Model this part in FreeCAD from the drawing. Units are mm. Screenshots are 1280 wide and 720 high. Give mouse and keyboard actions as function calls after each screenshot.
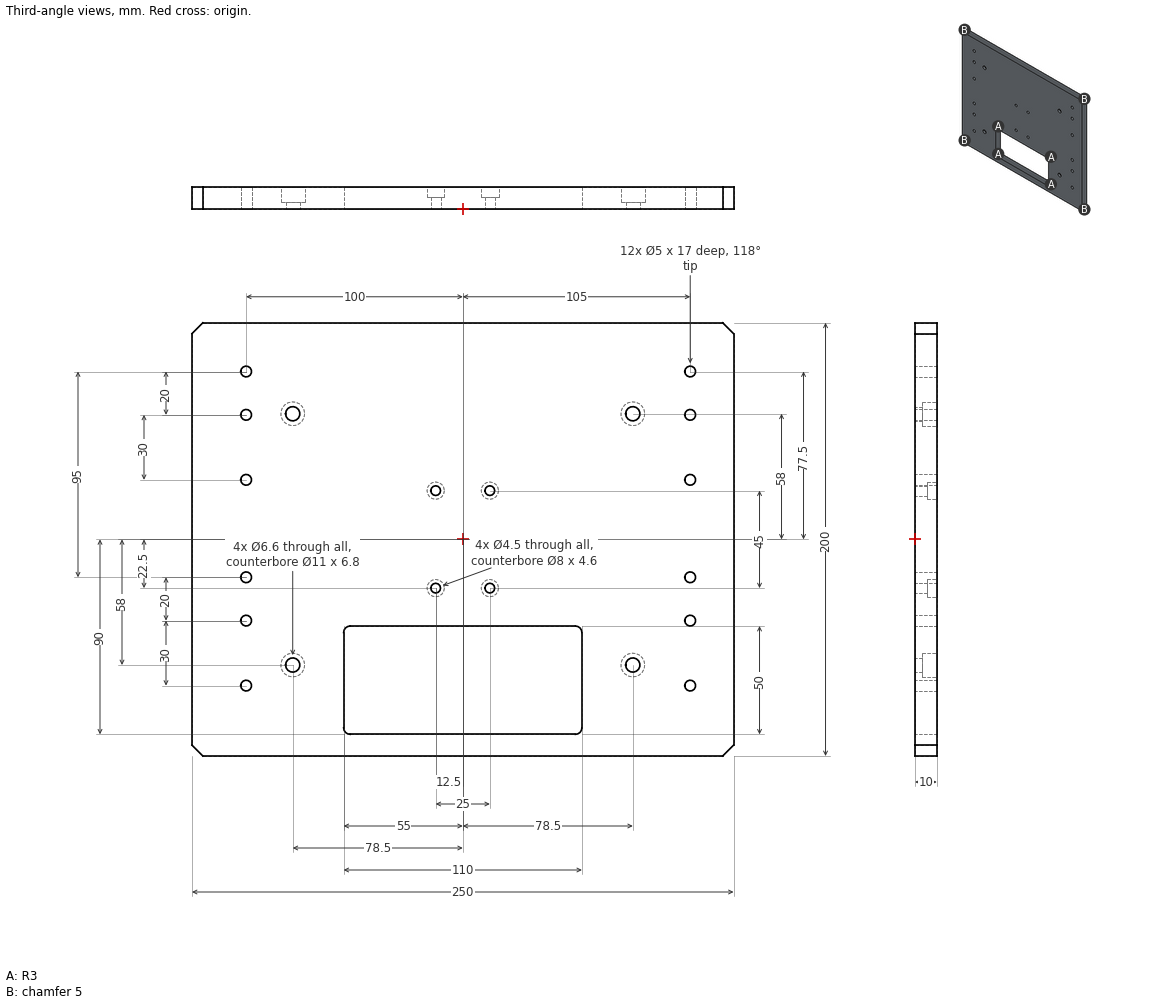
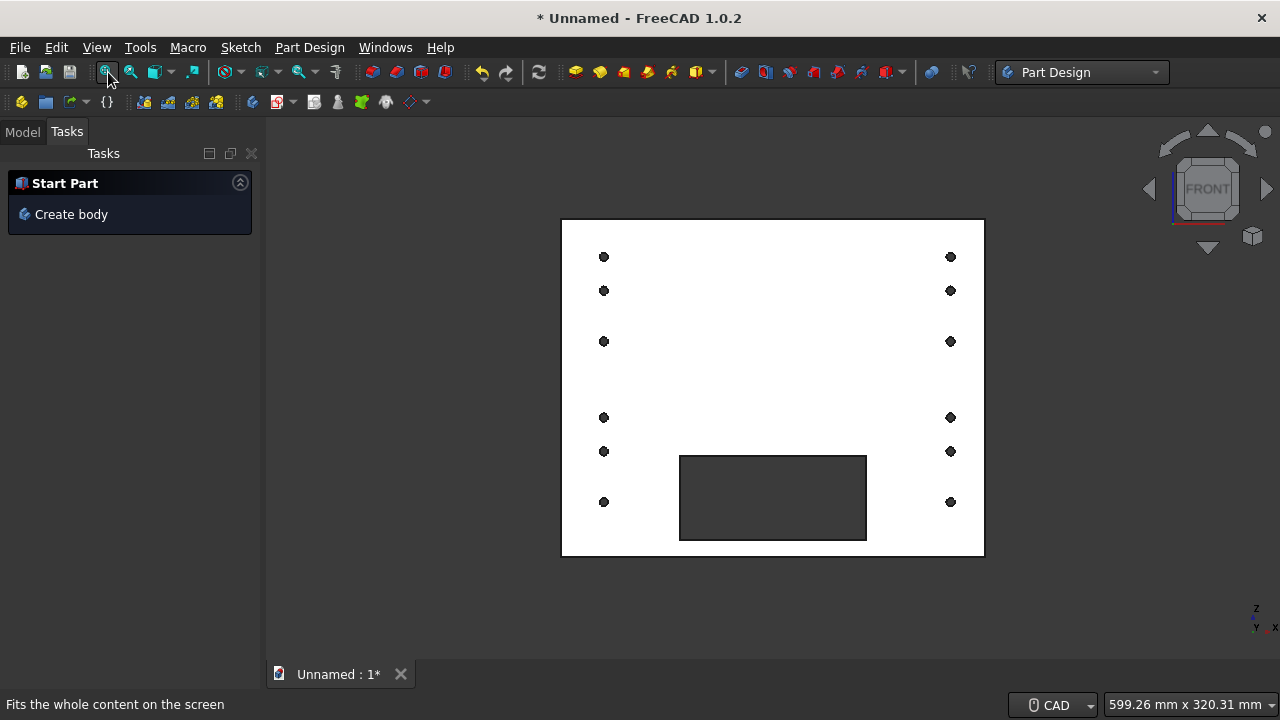
key(3)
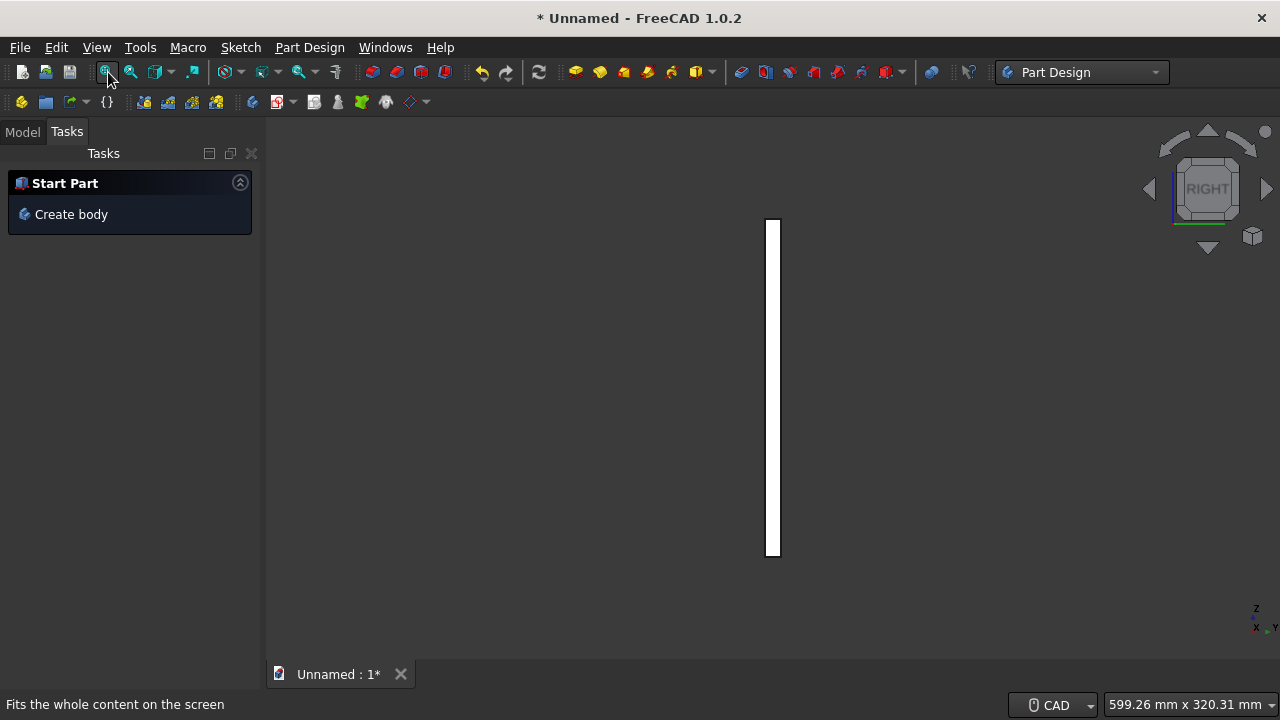
scroll(773, 455, up, 5)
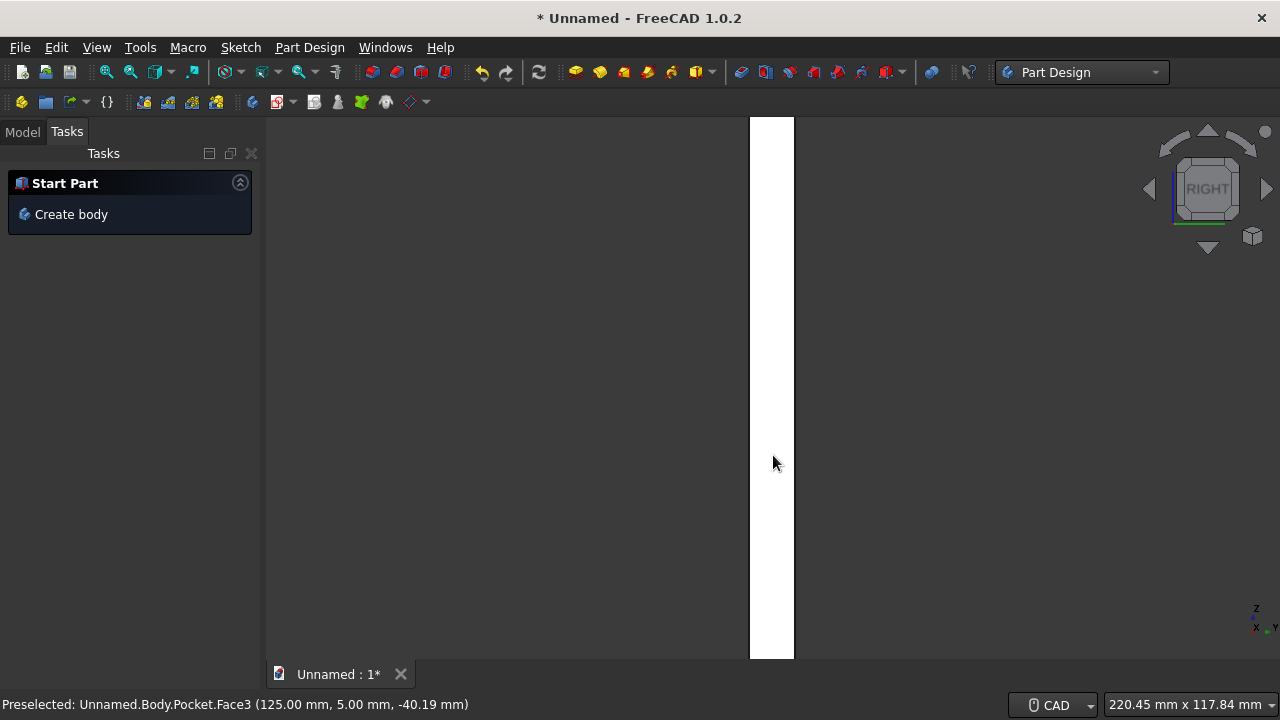
click(108, 72)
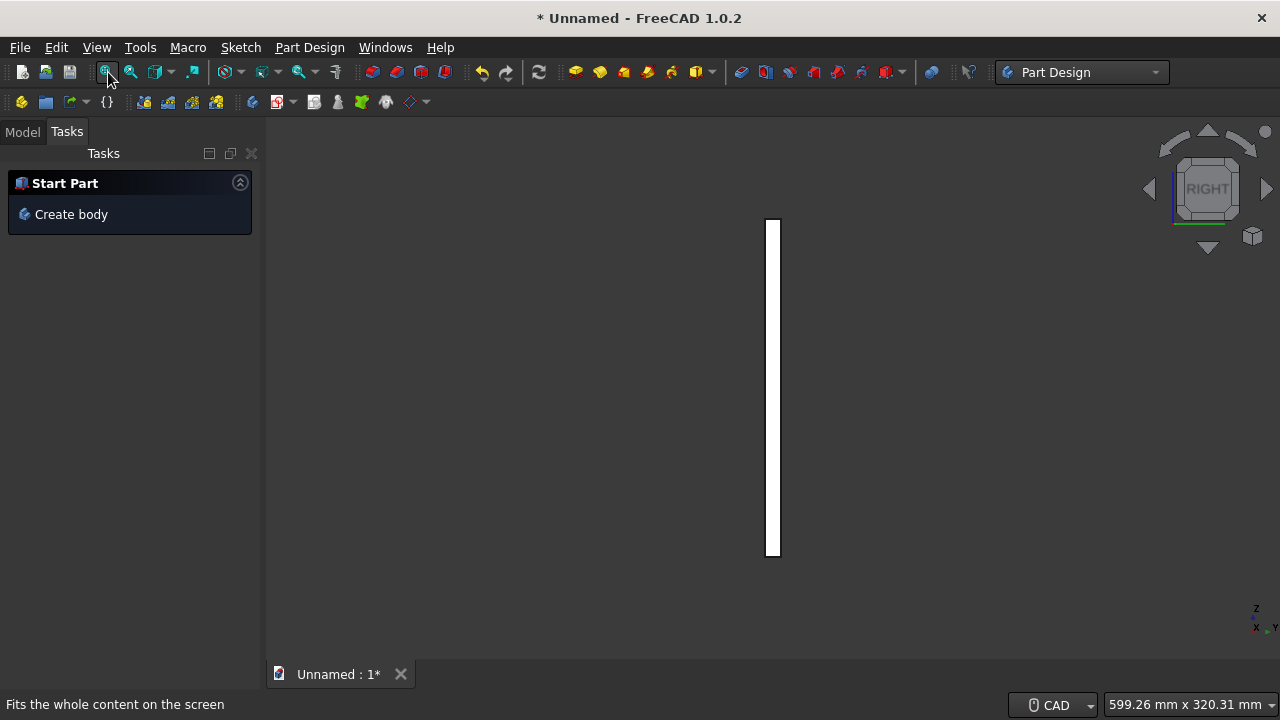
key(5)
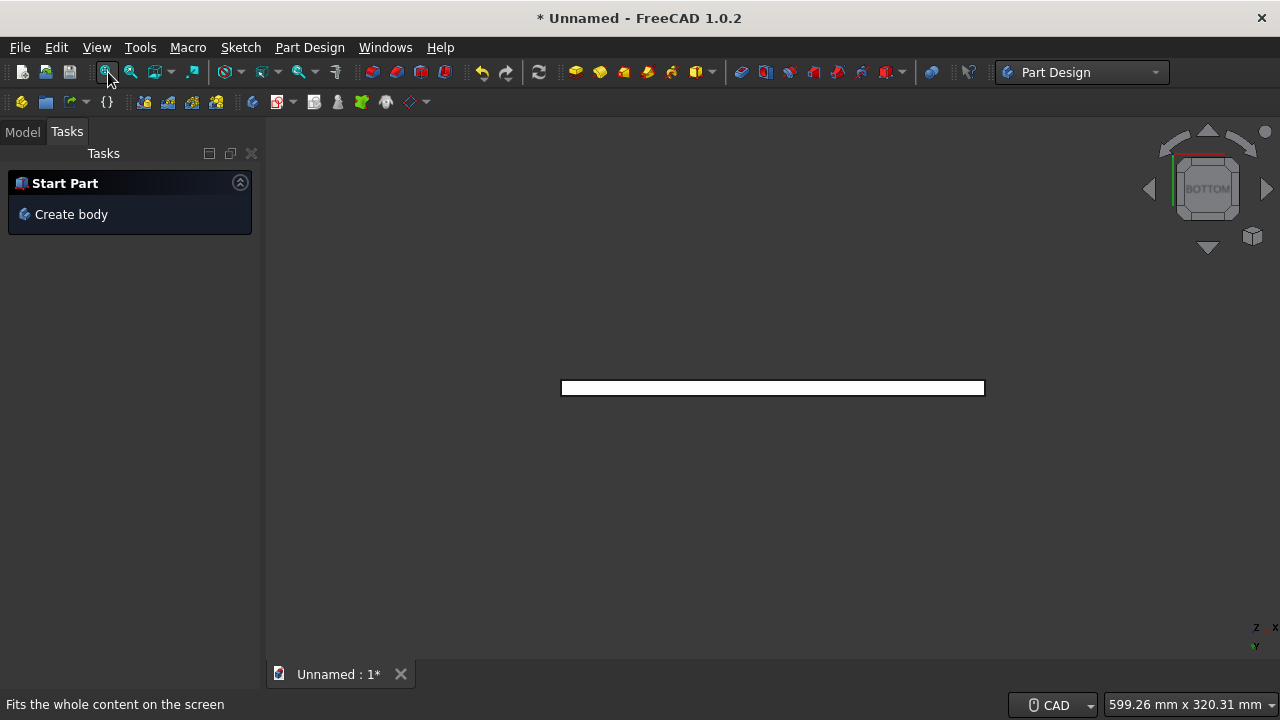
click(108, 72)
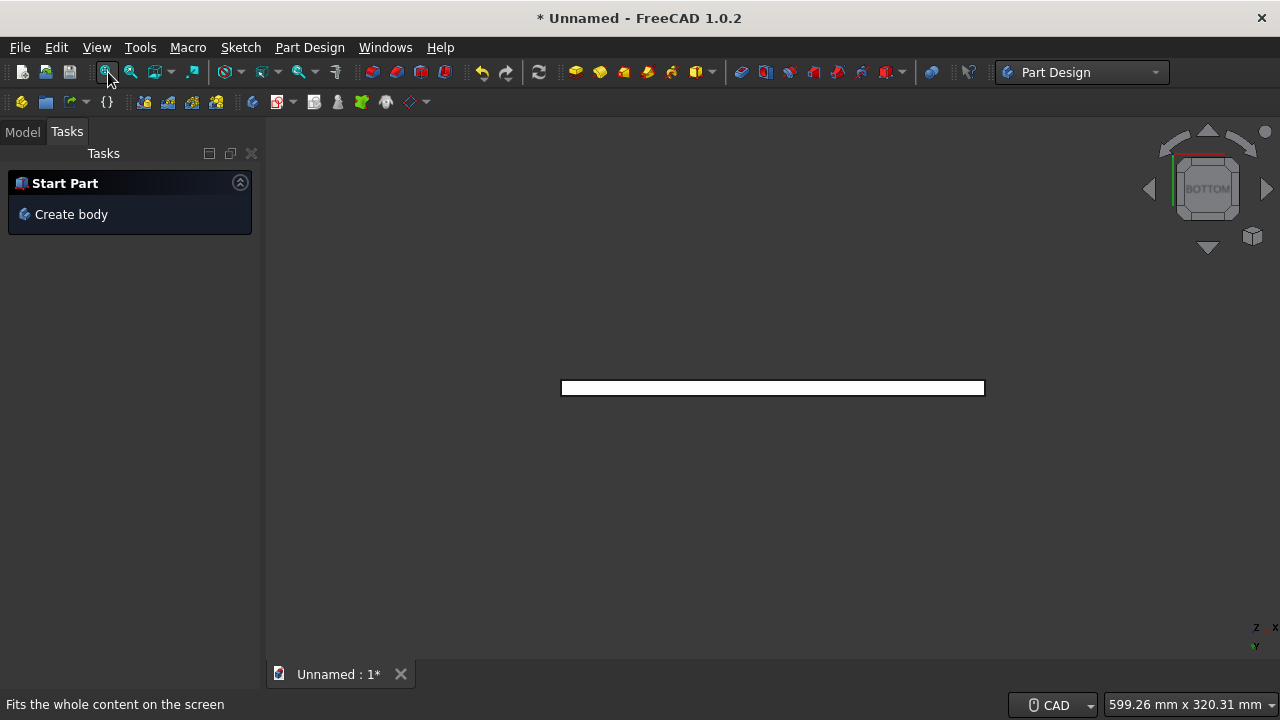
scroll(680, 387, up, 5)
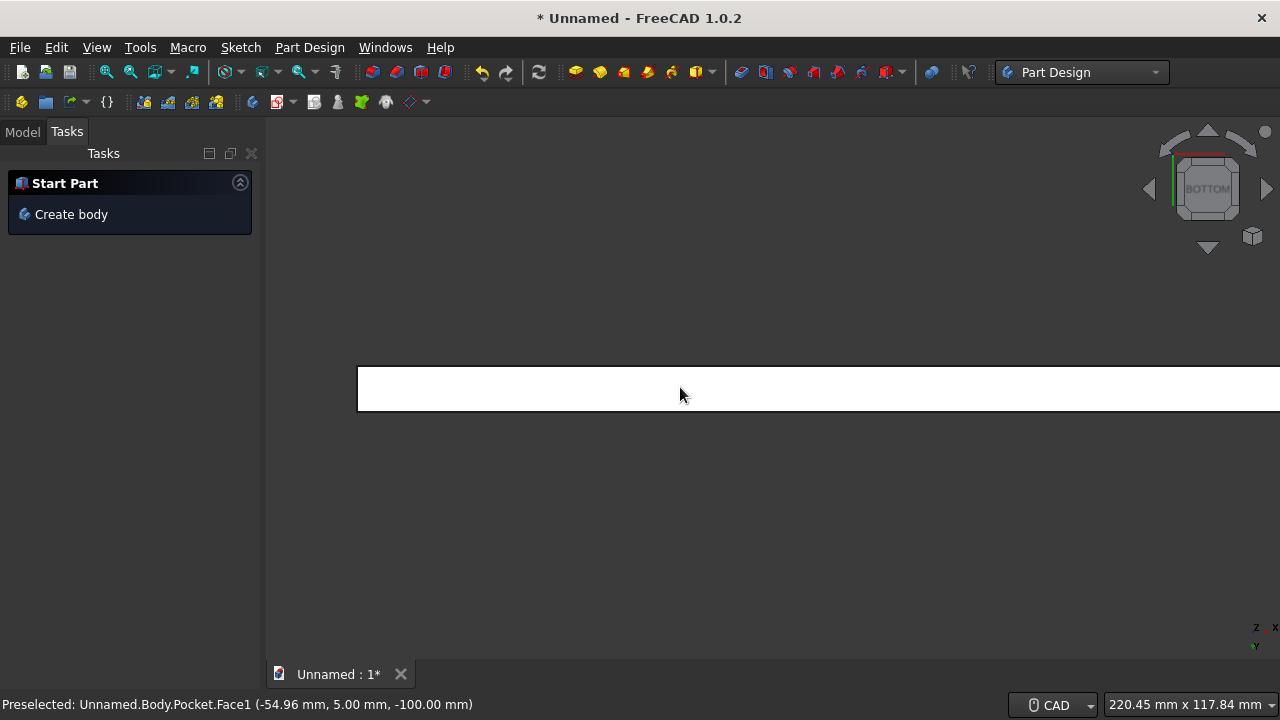
click(108, 72)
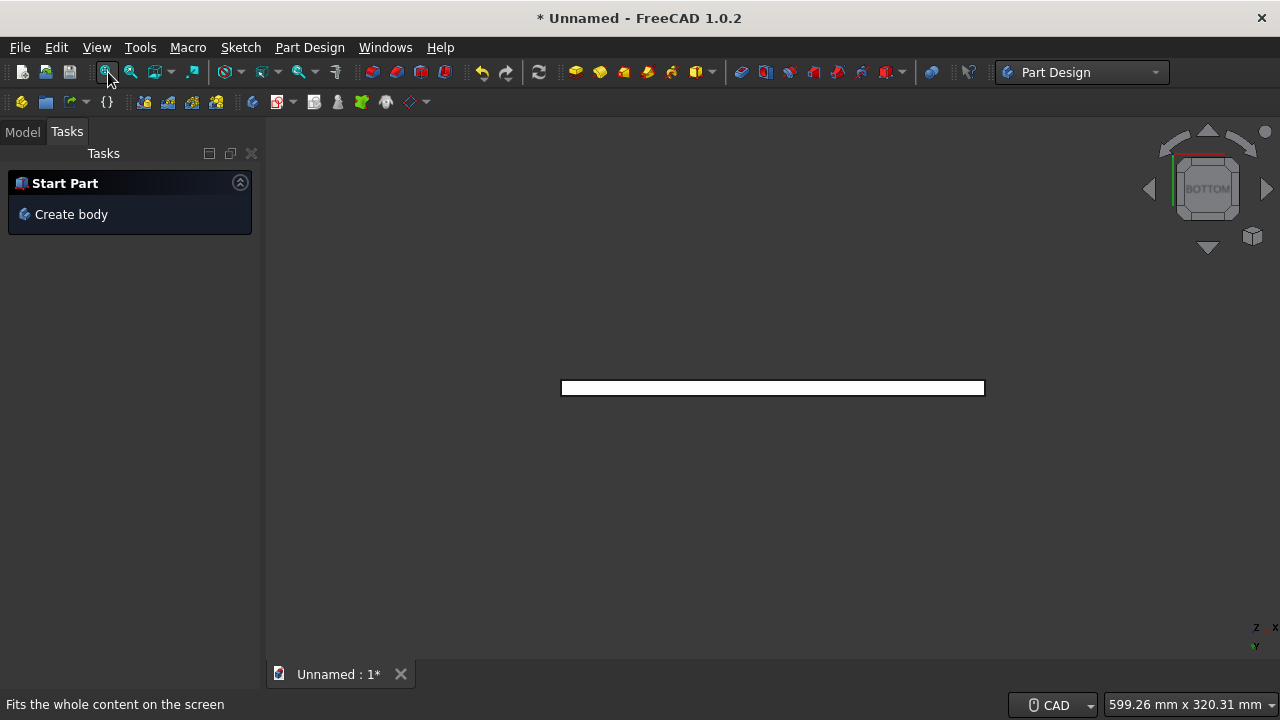
key(4)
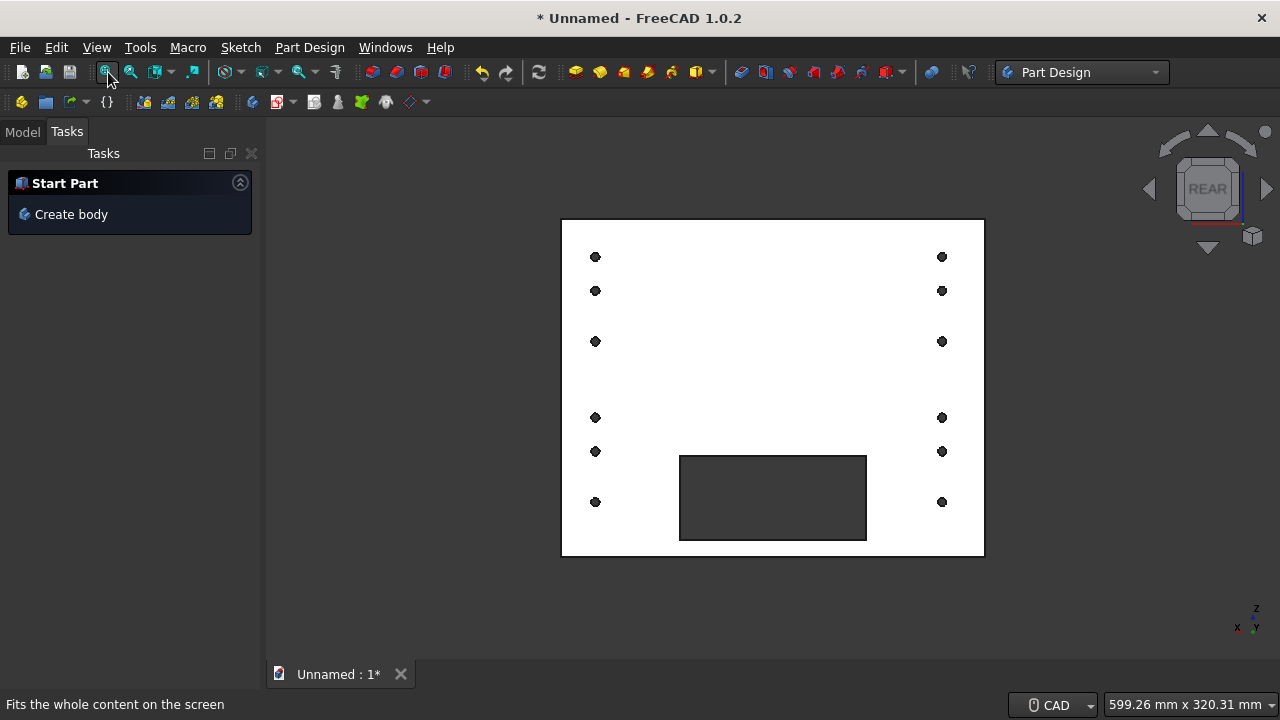
scroll(866, 455, up, 5)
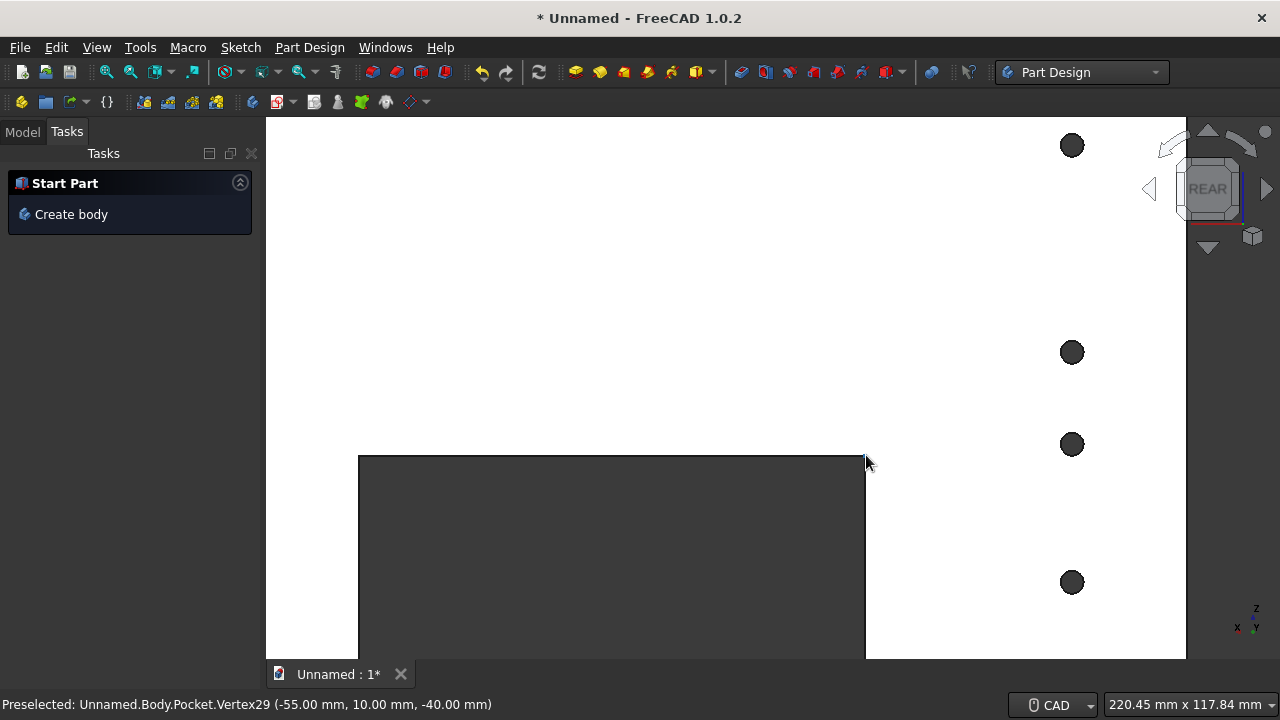
click(108, 72)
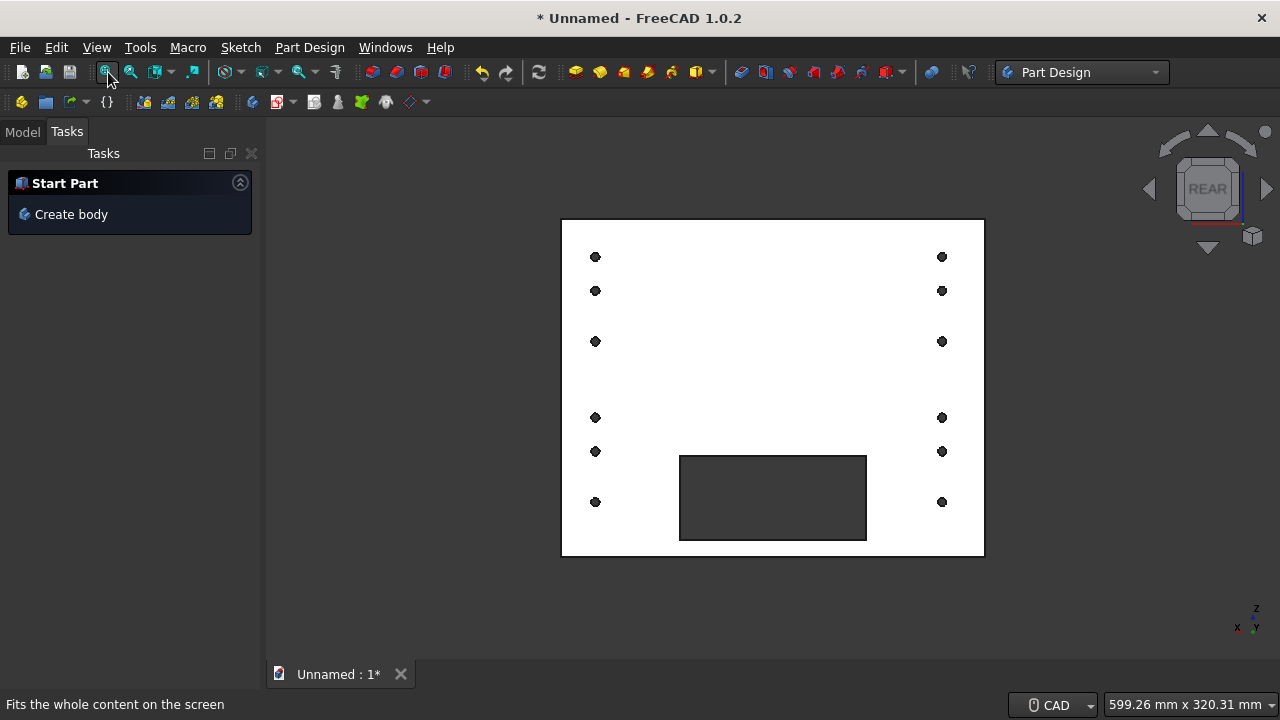
key(6)